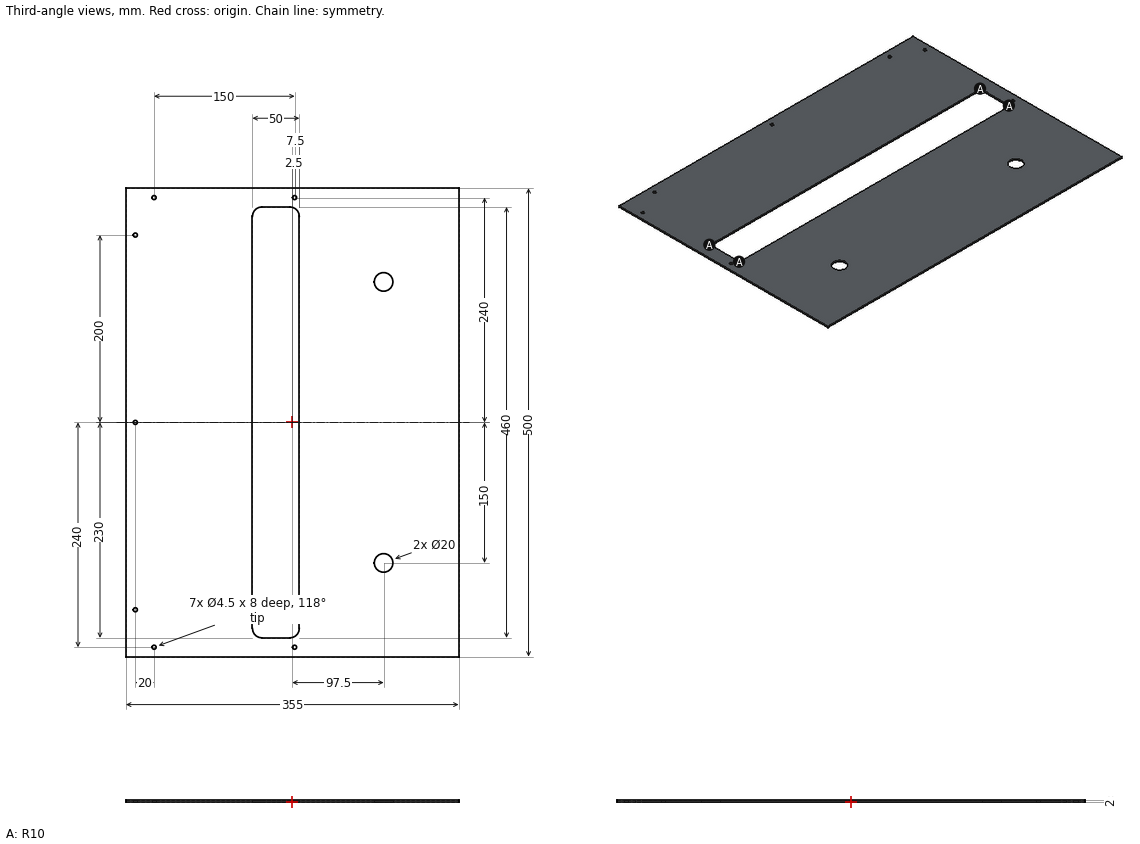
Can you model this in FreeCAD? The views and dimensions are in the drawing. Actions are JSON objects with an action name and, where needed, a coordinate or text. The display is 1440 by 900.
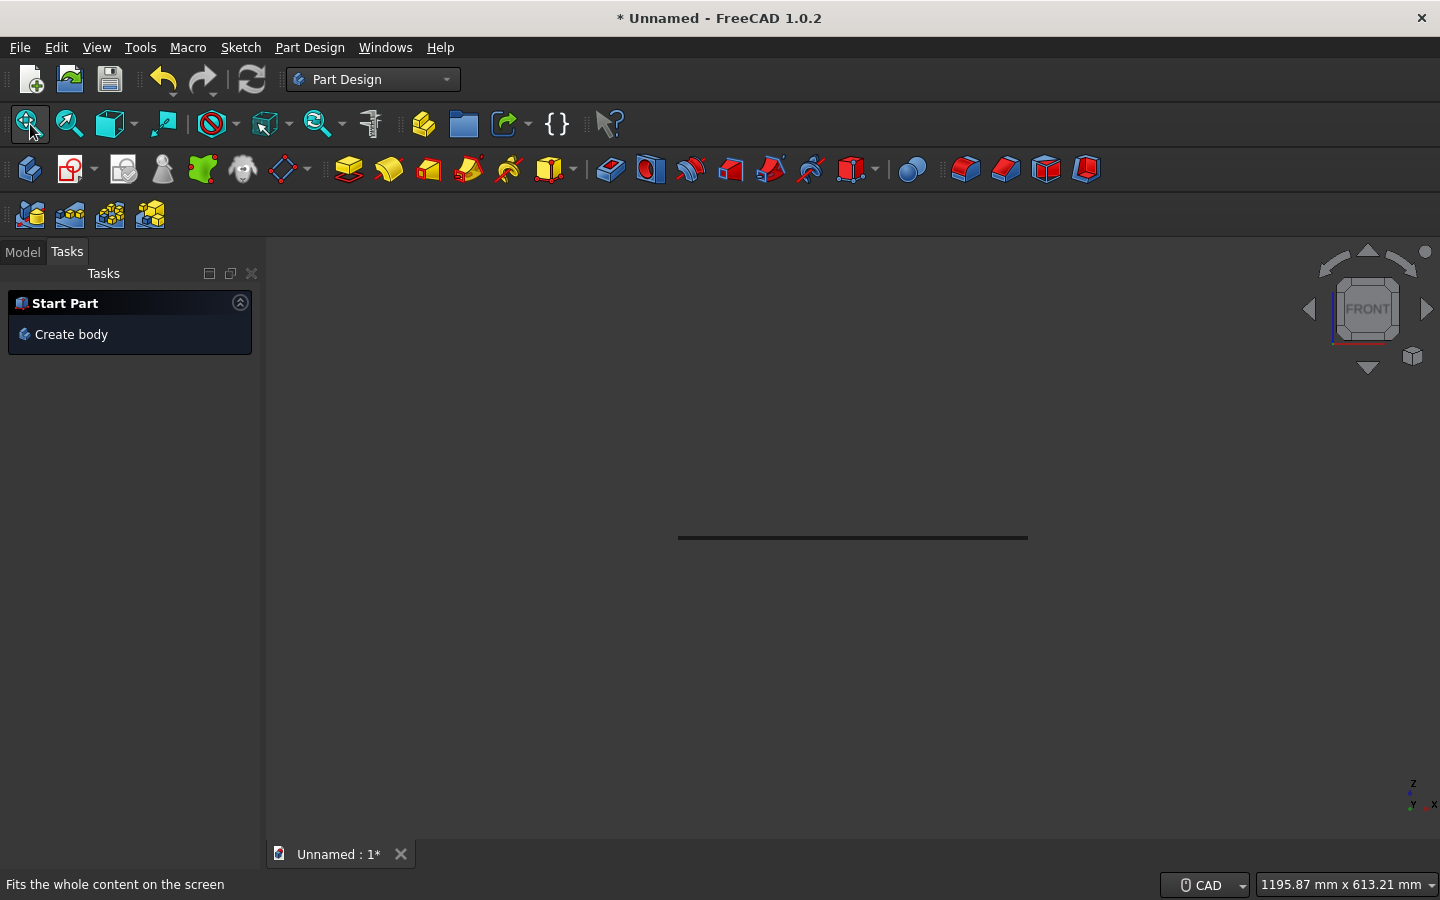
{"action": "left_click", "coordinate": [30, 124]}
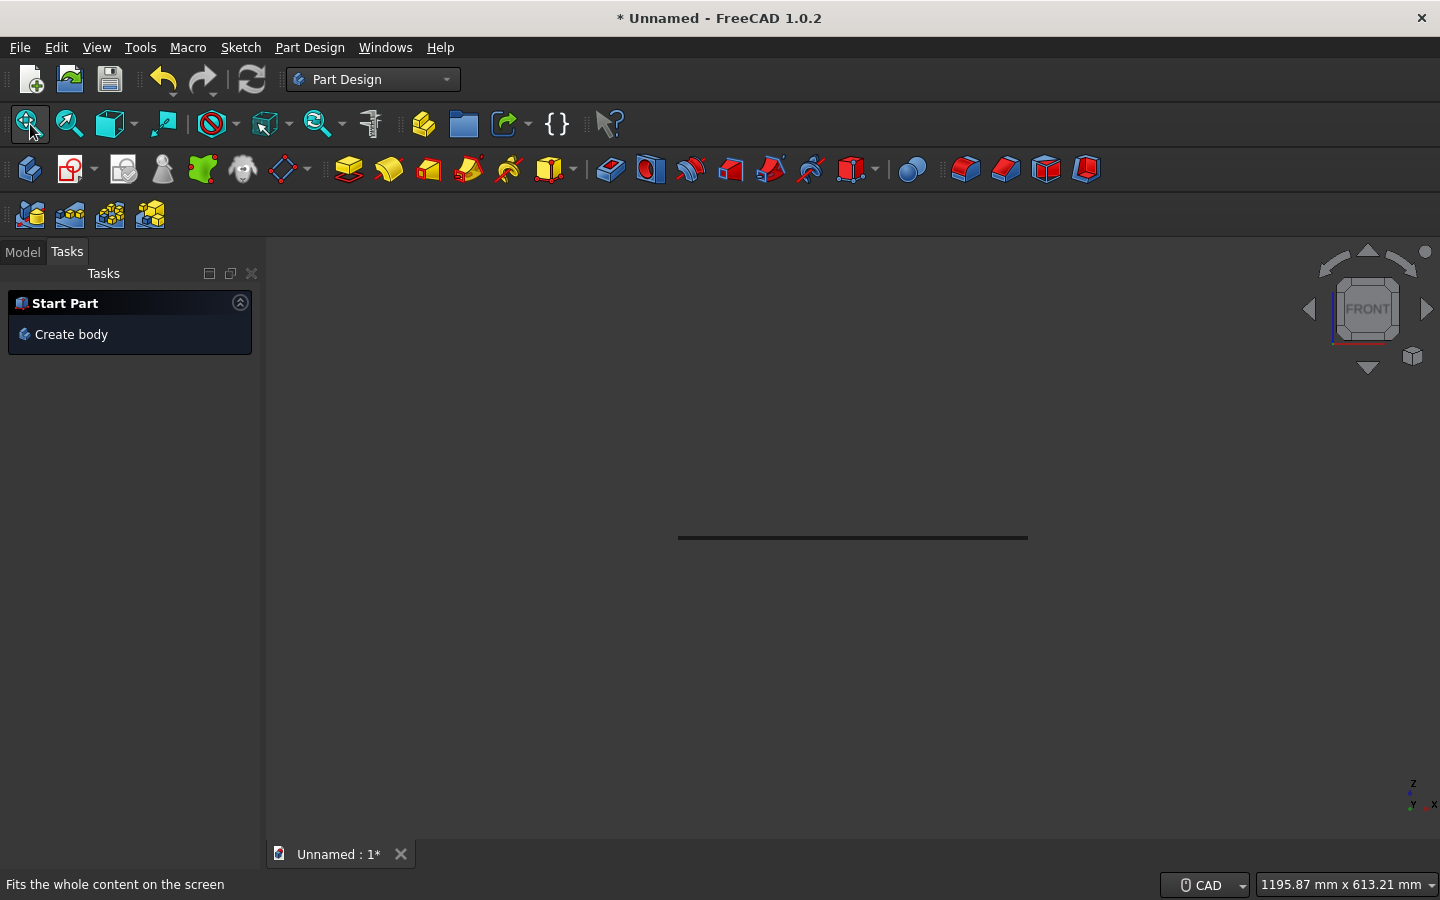
{"action": "scroll", "coordinate": [811, 537], "scroll_direction": "up", "scroll_amount": 15}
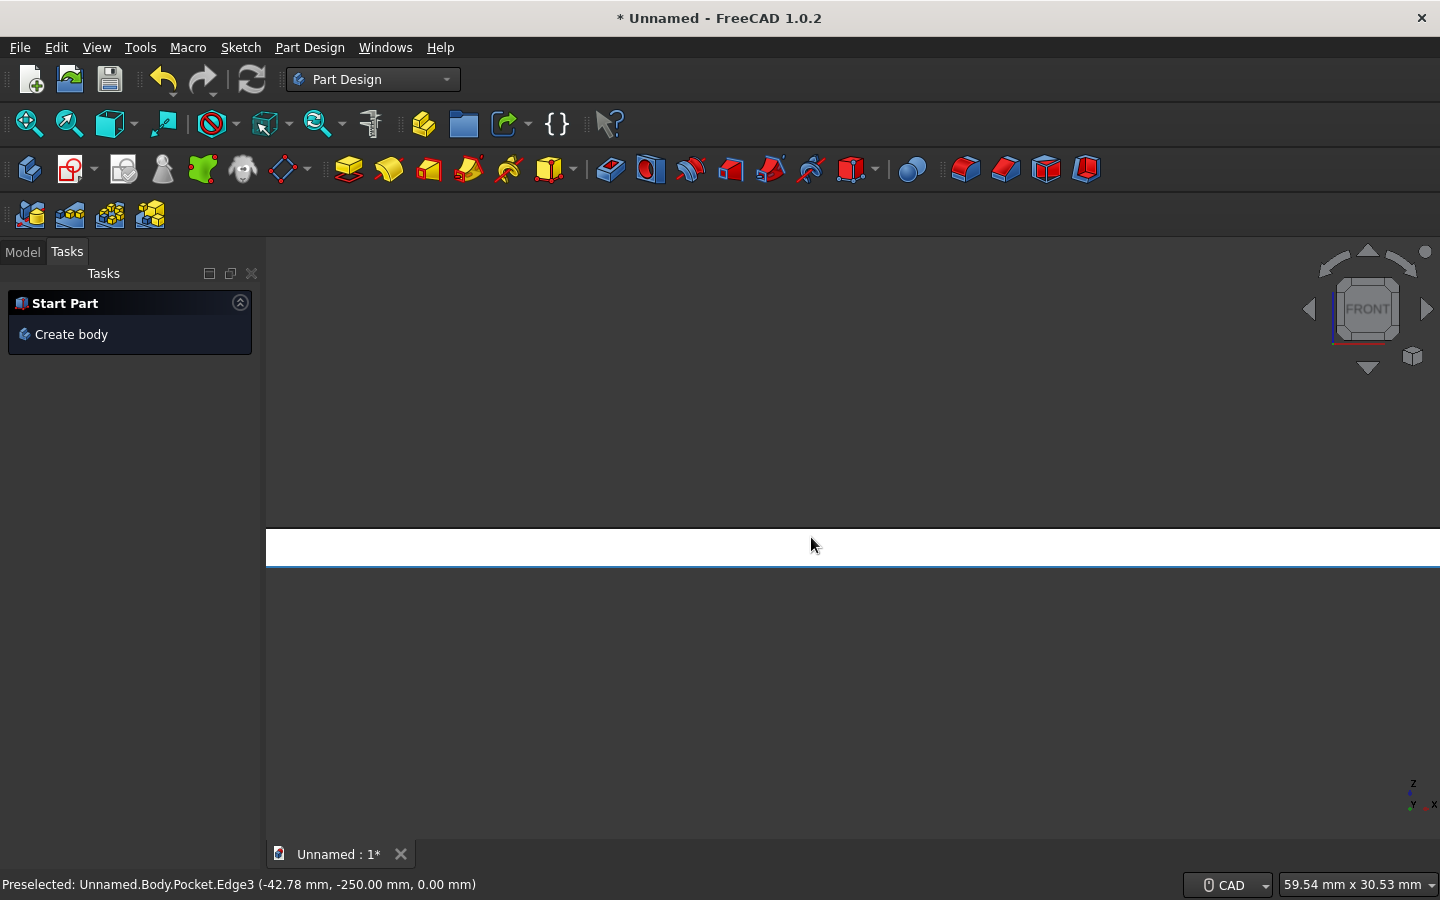
{"action": "key", "text": "v f"}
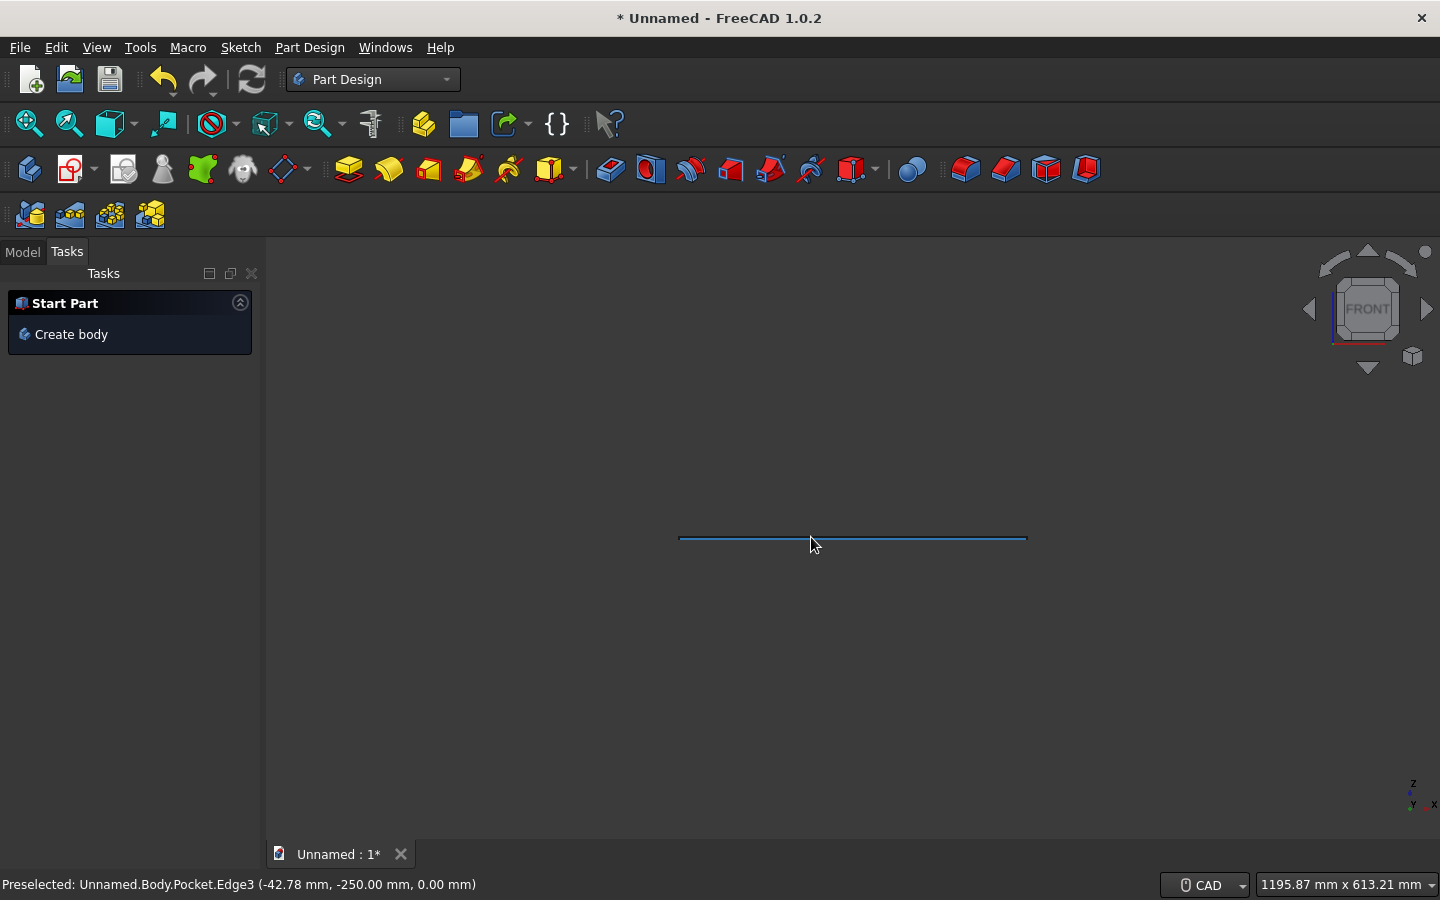
{"action": "key", "text": "3"}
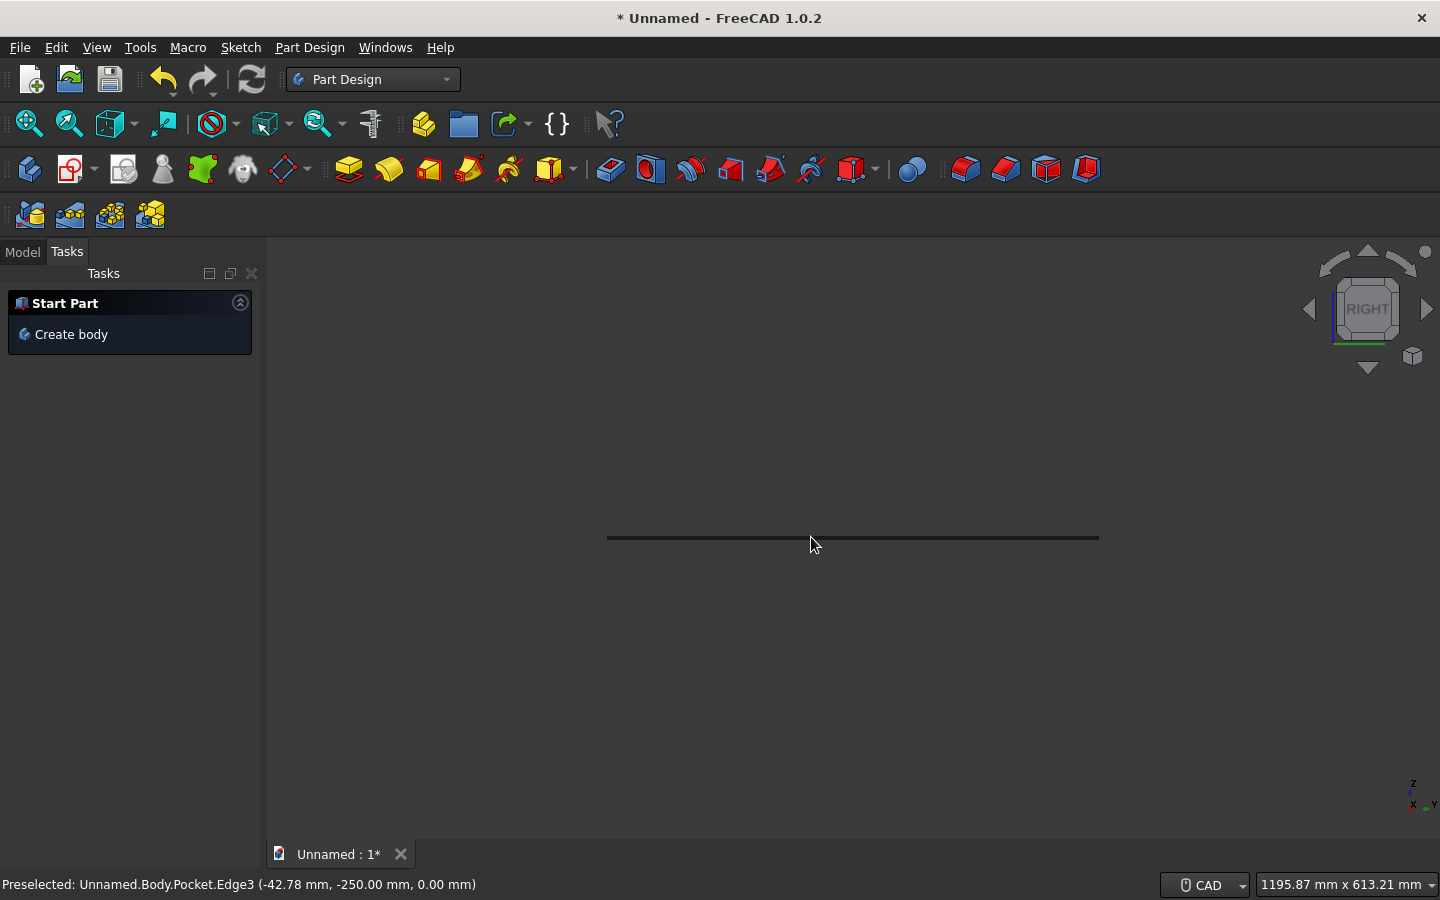
{"action": "left_click", "coordinate": [30, 124]}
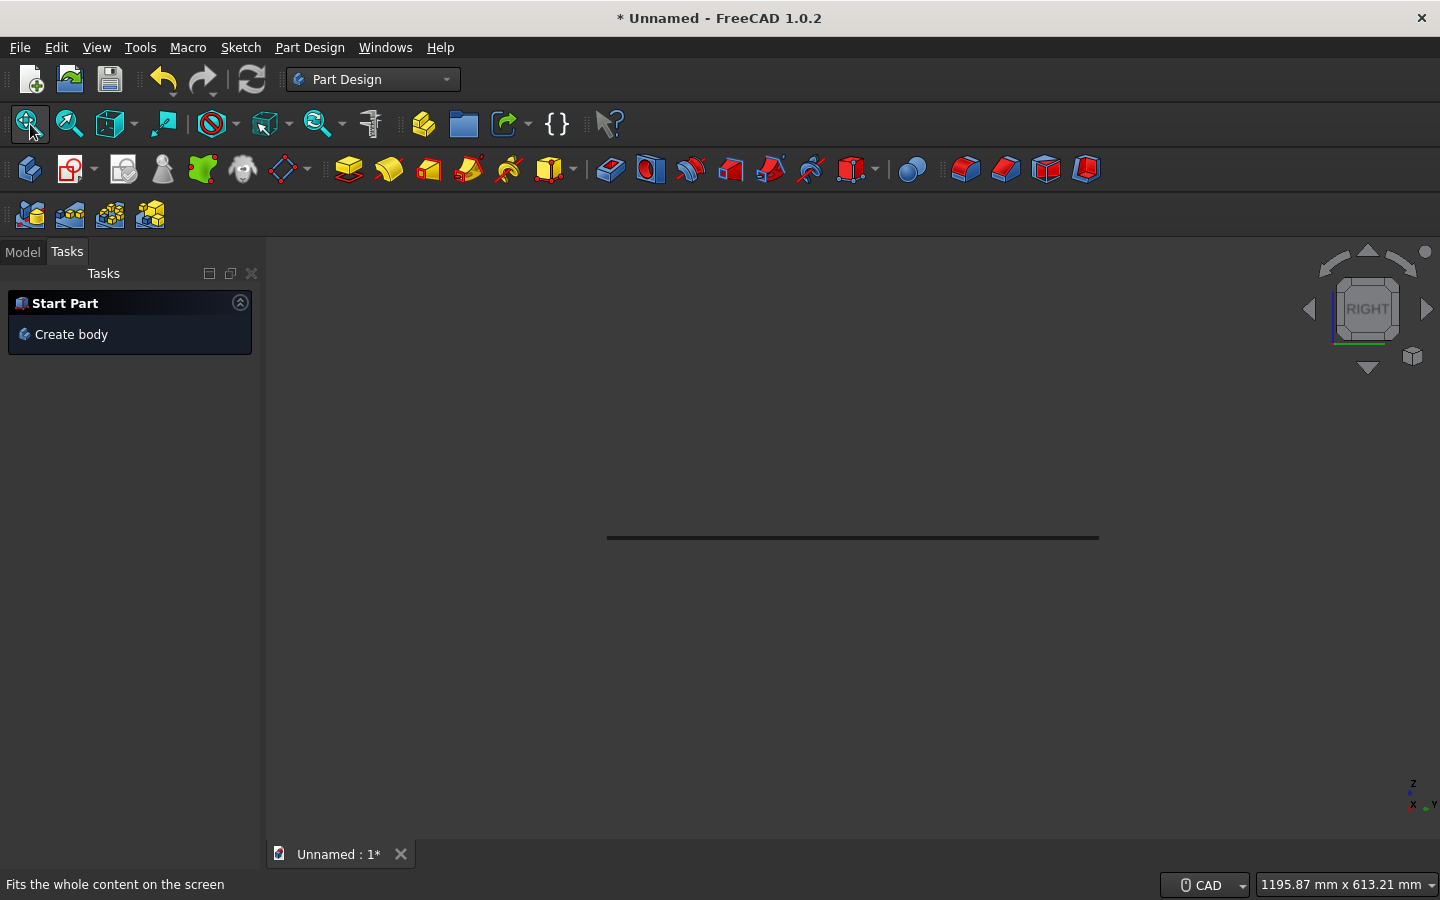
{"action": "scroll", "coordinate": [1079, 537], "scroll_direction": "up", "scroll_amount": 15}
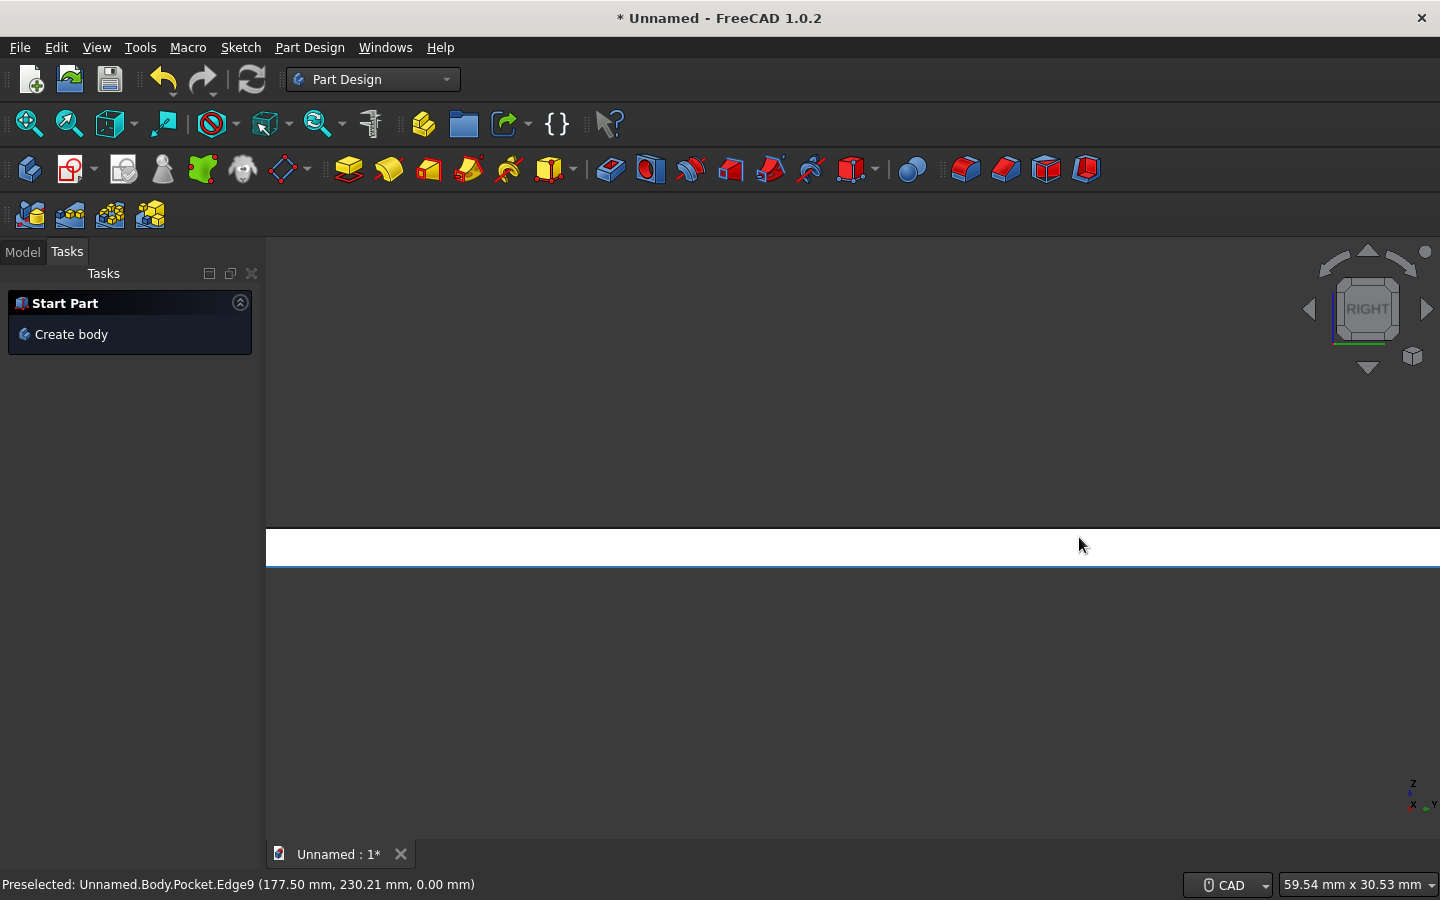
{"action": "left_click", "coordinate": [30, 124]}